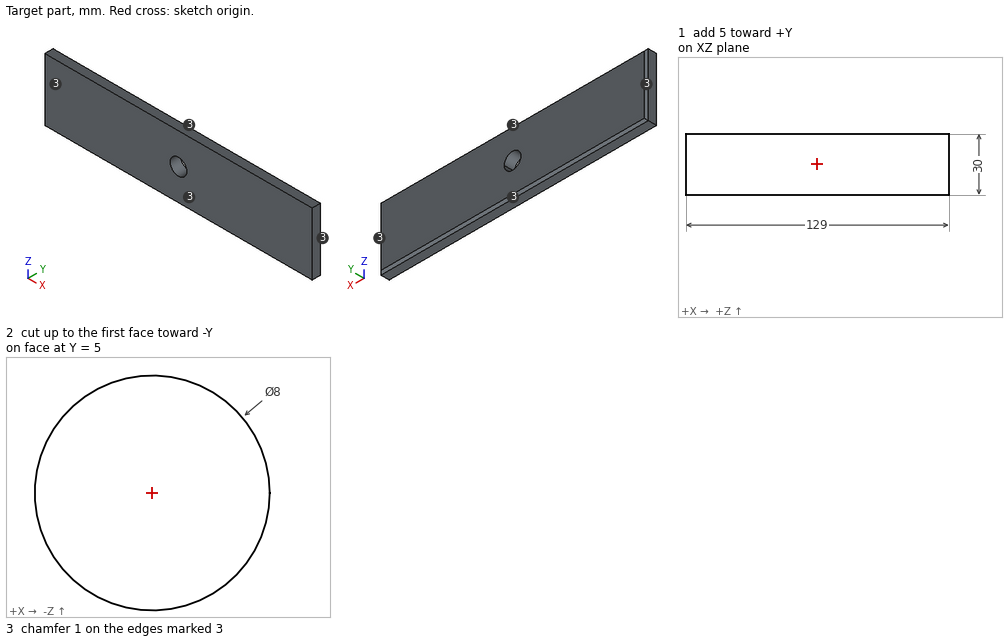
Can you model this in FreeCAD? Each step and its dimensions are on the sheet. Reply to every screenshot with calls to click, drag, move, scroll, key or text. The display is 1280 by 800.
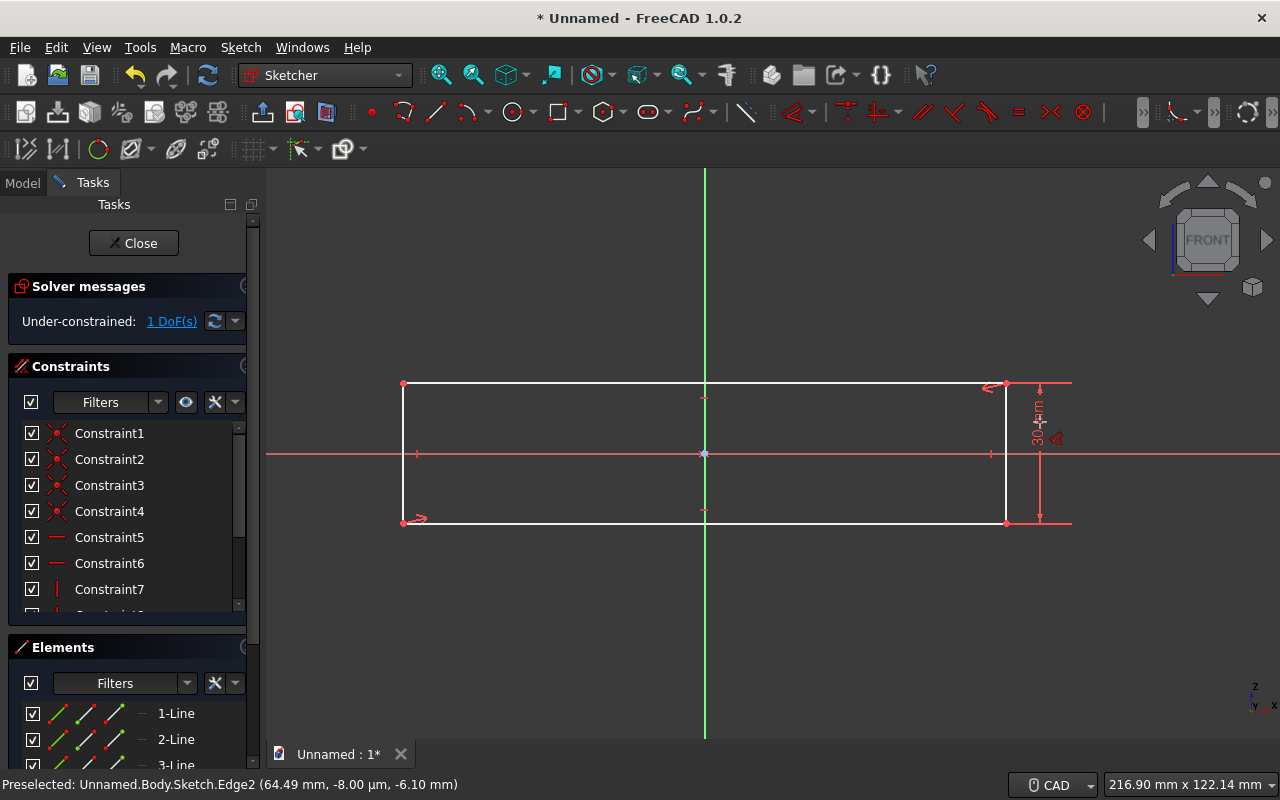
click(584, 524)
click(566, 558)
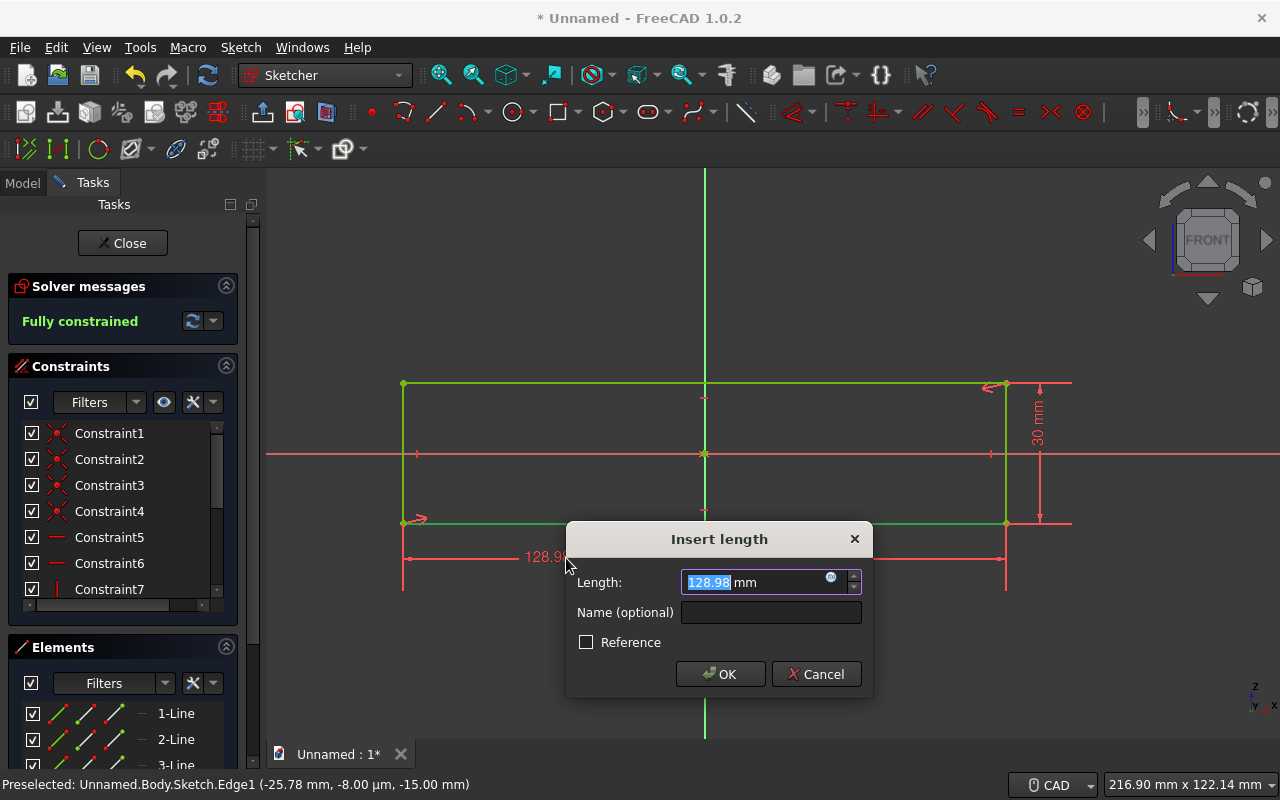
text(129)
key(Return)
key(Escape)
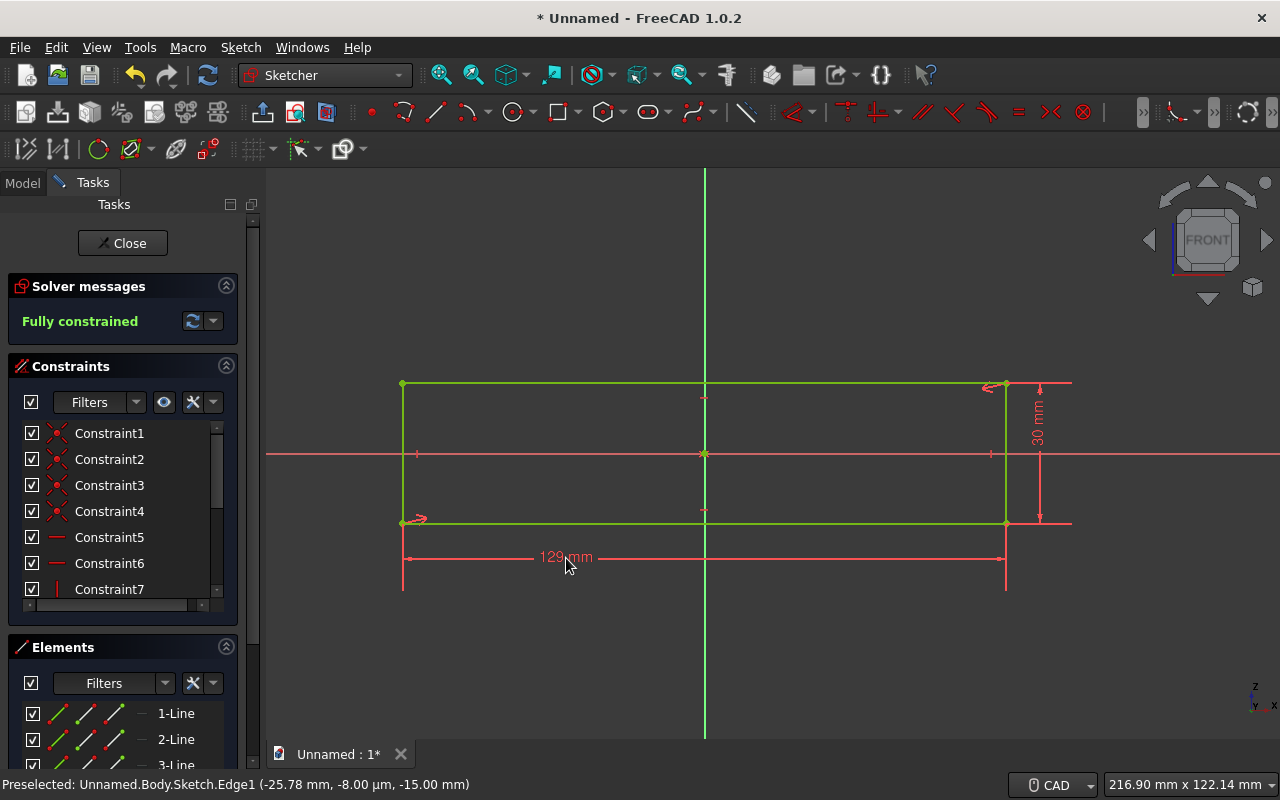
click(123, 243)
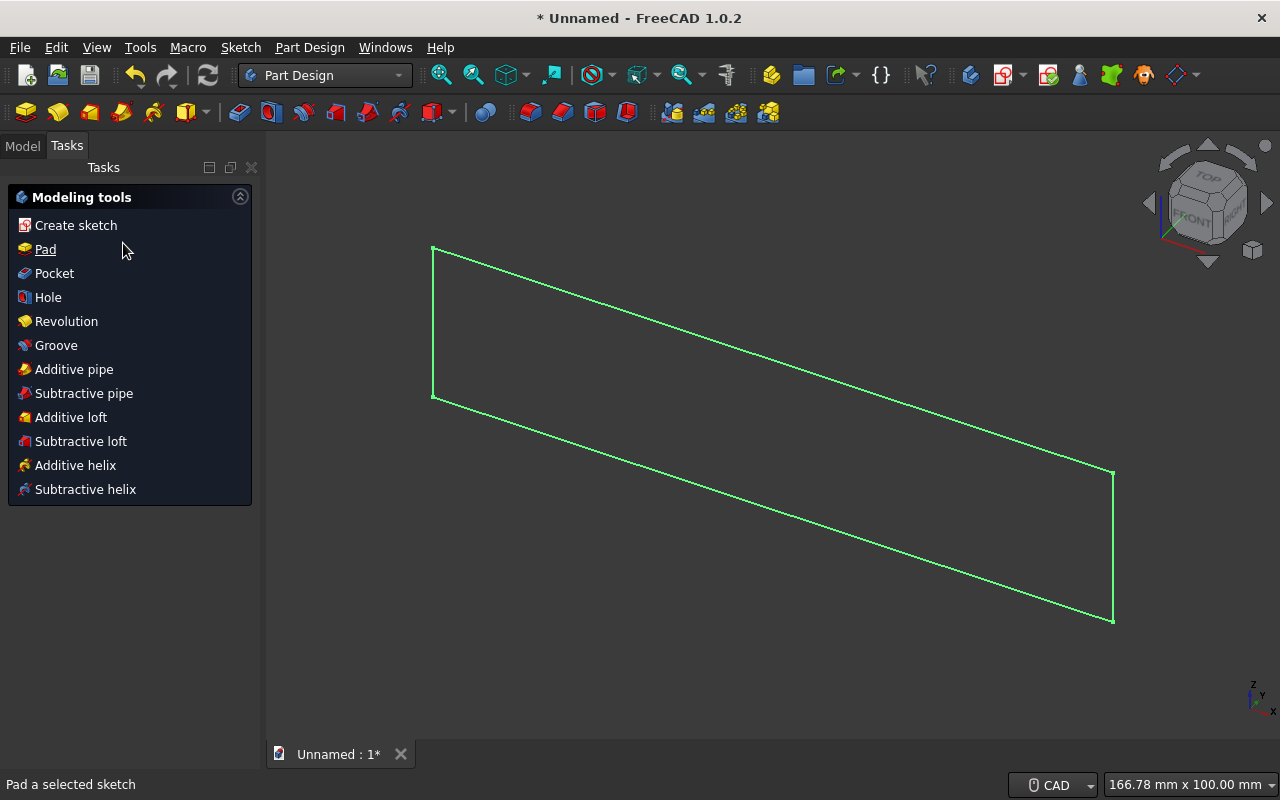
click(26, 112)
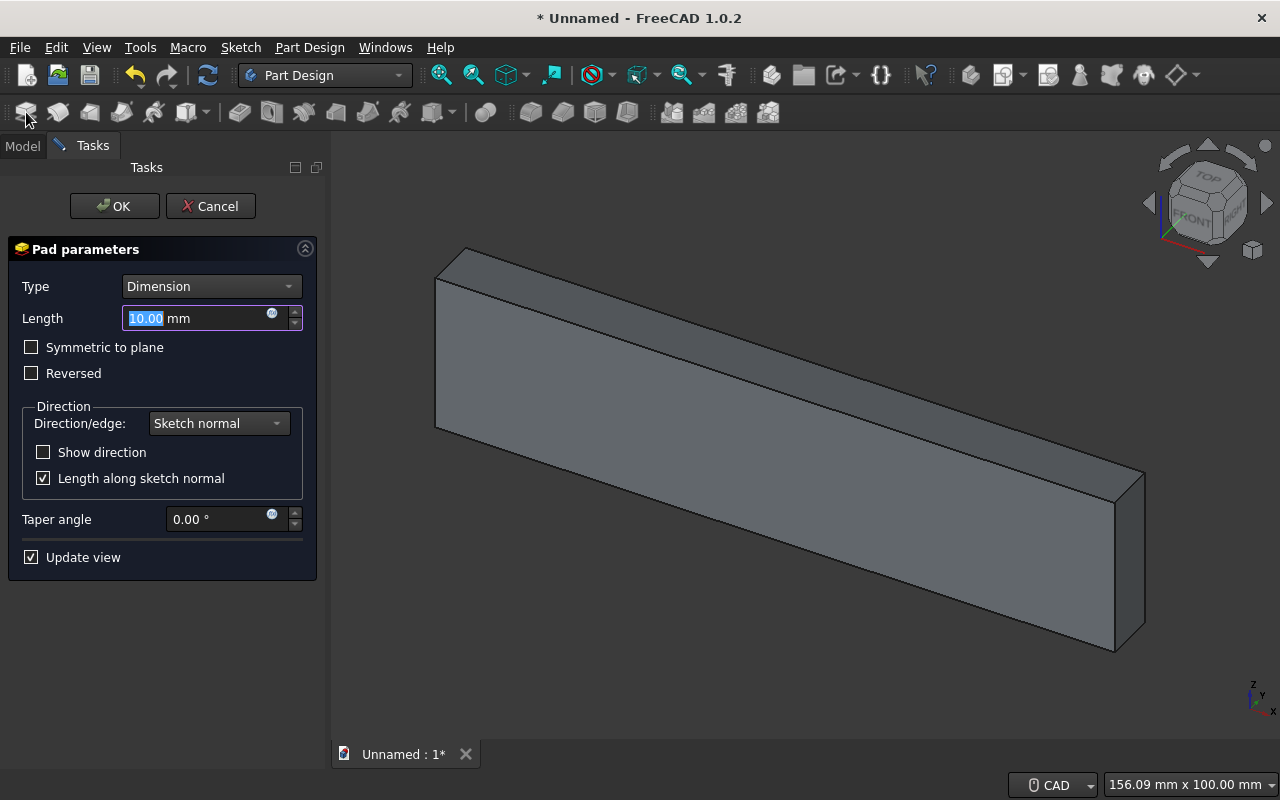
text(5)
key(Tab)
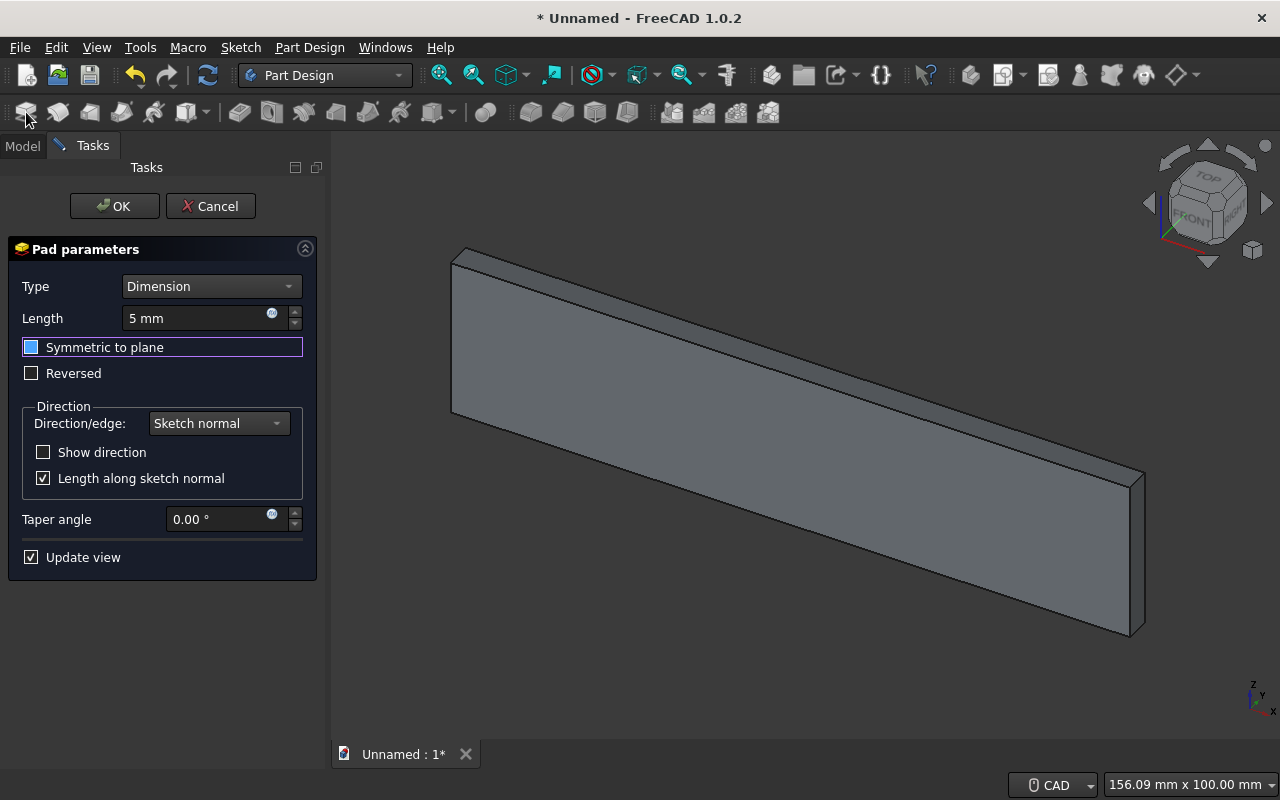
click(30, 373)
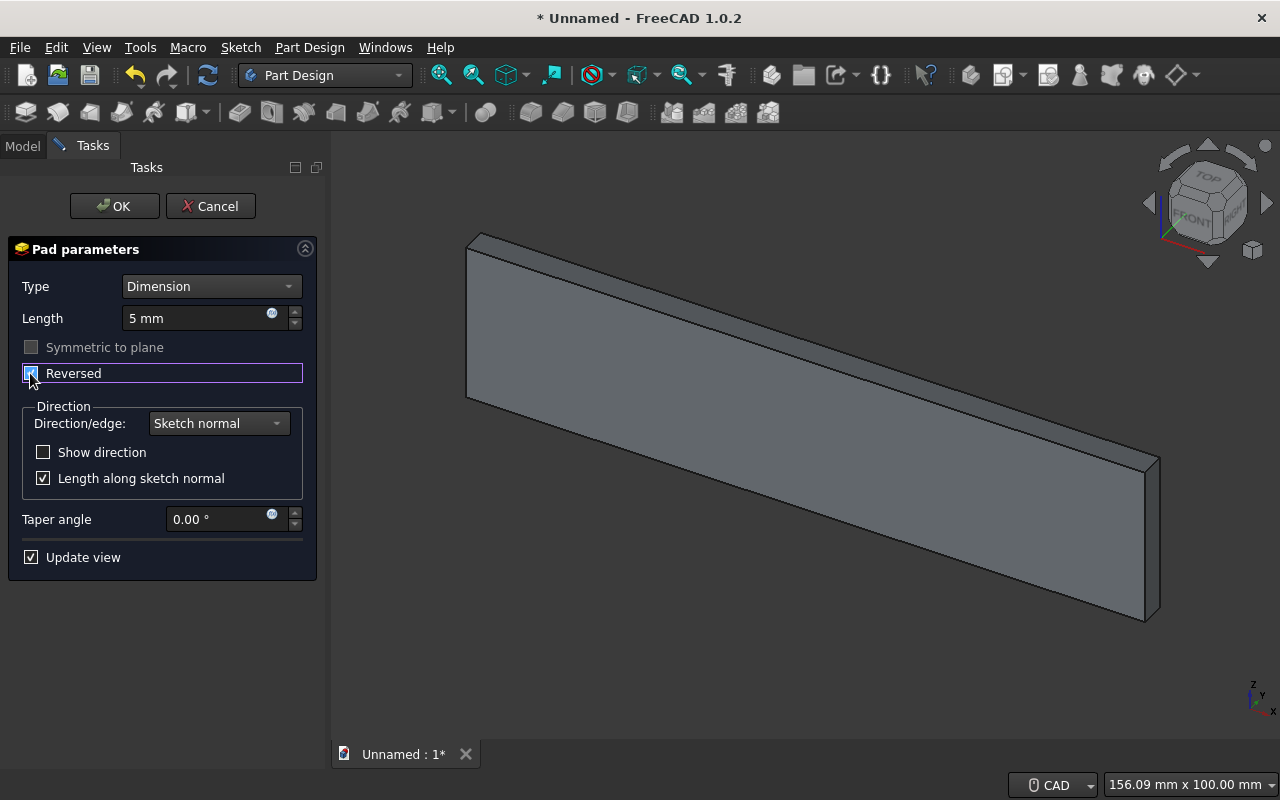
click(115, 206)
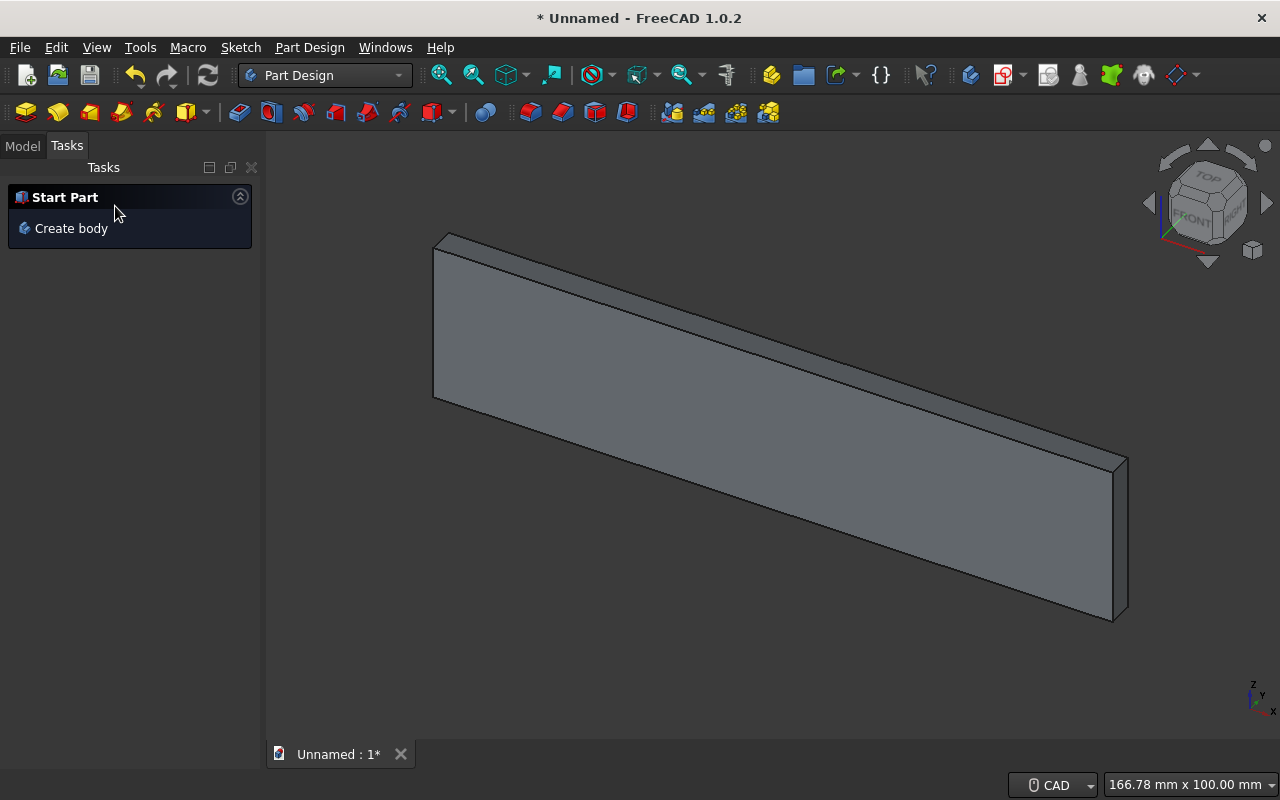
key(4)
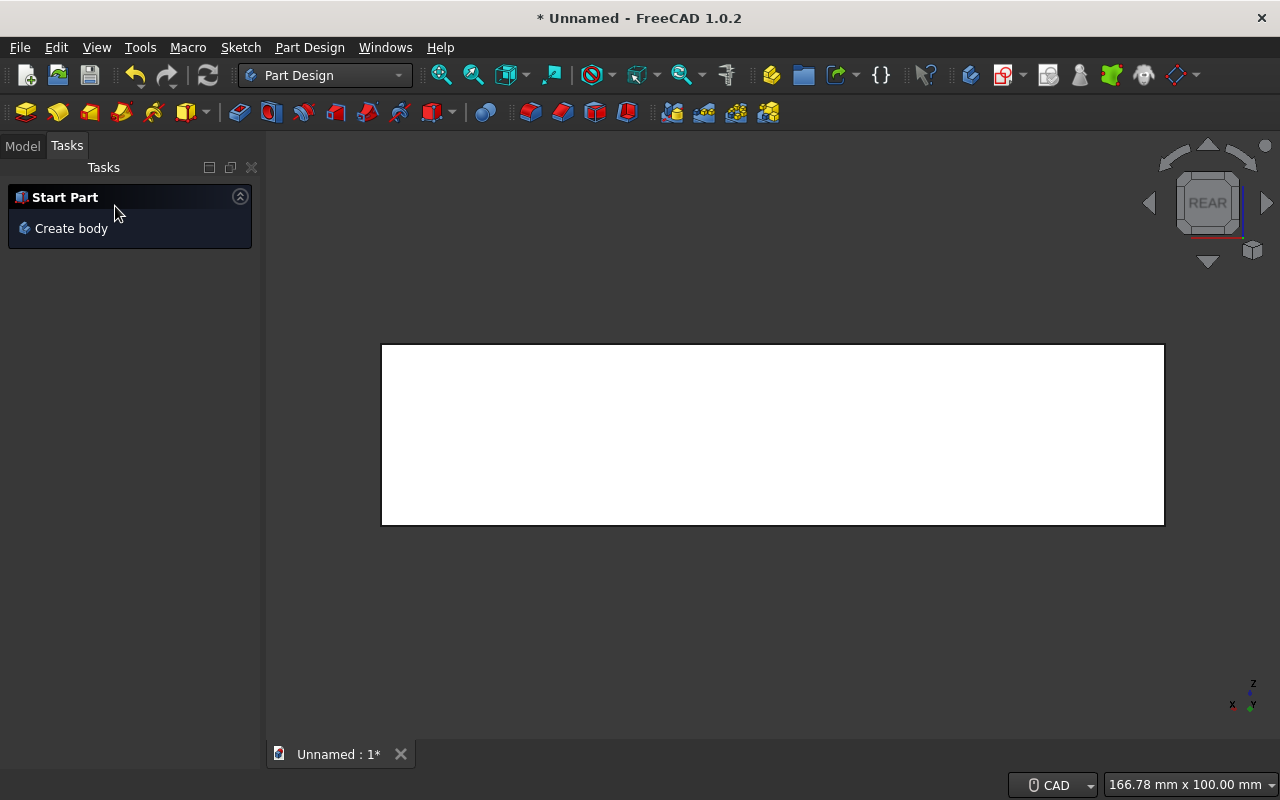
click(549, 434)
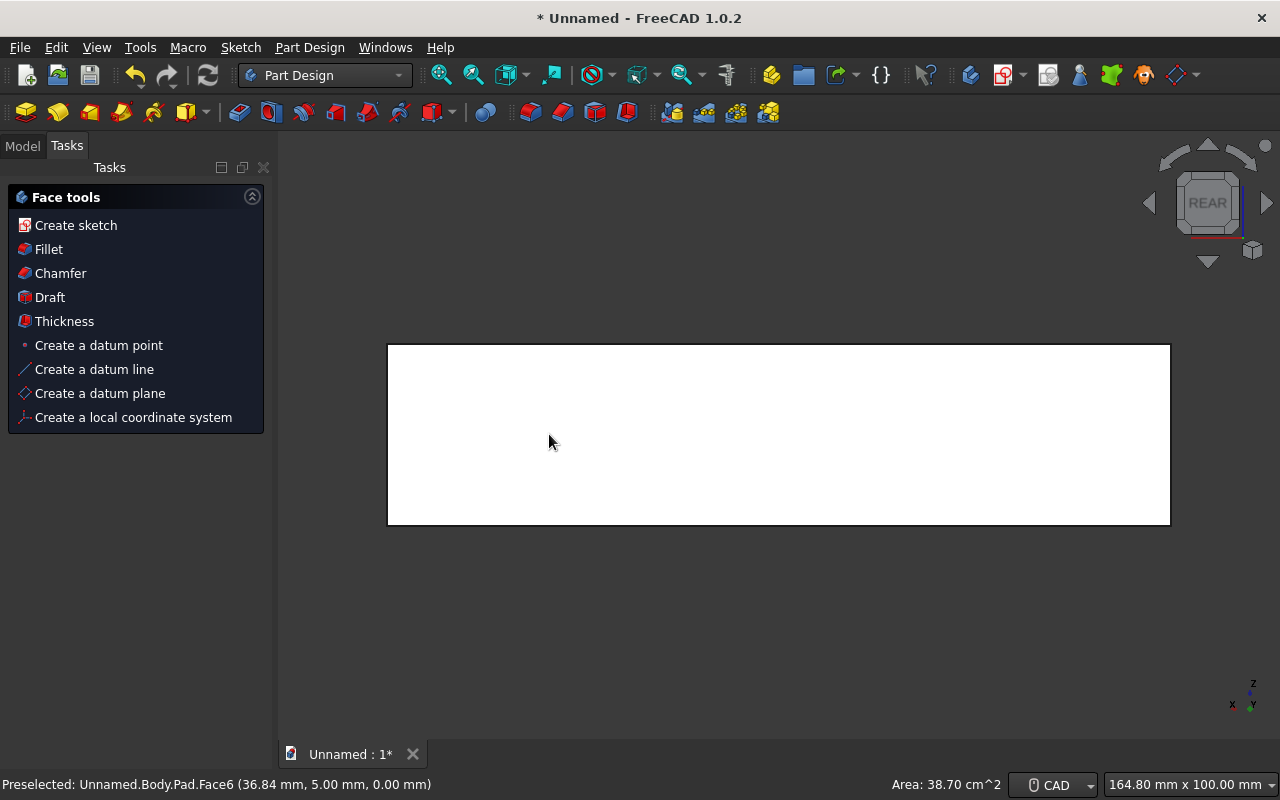
click(1004, 76)